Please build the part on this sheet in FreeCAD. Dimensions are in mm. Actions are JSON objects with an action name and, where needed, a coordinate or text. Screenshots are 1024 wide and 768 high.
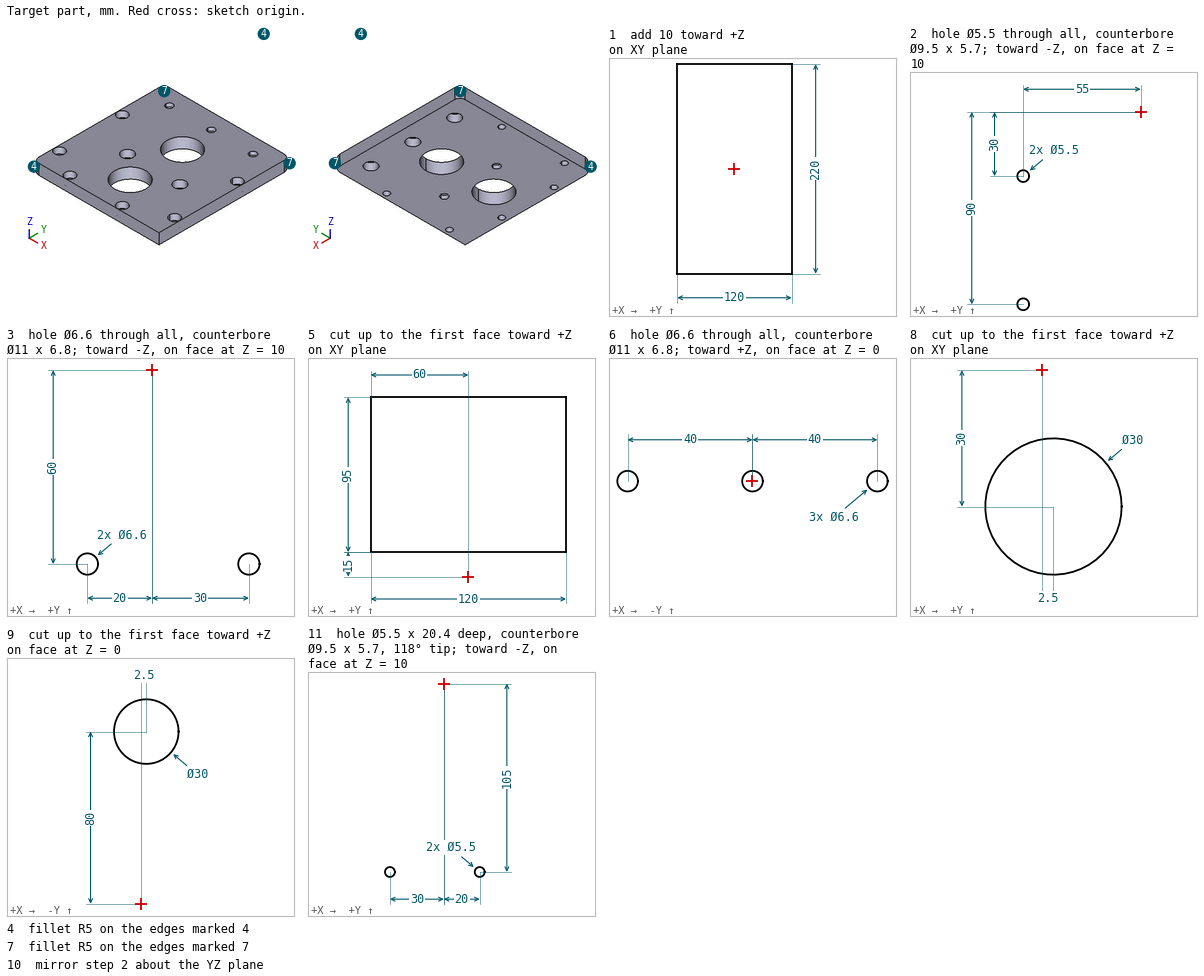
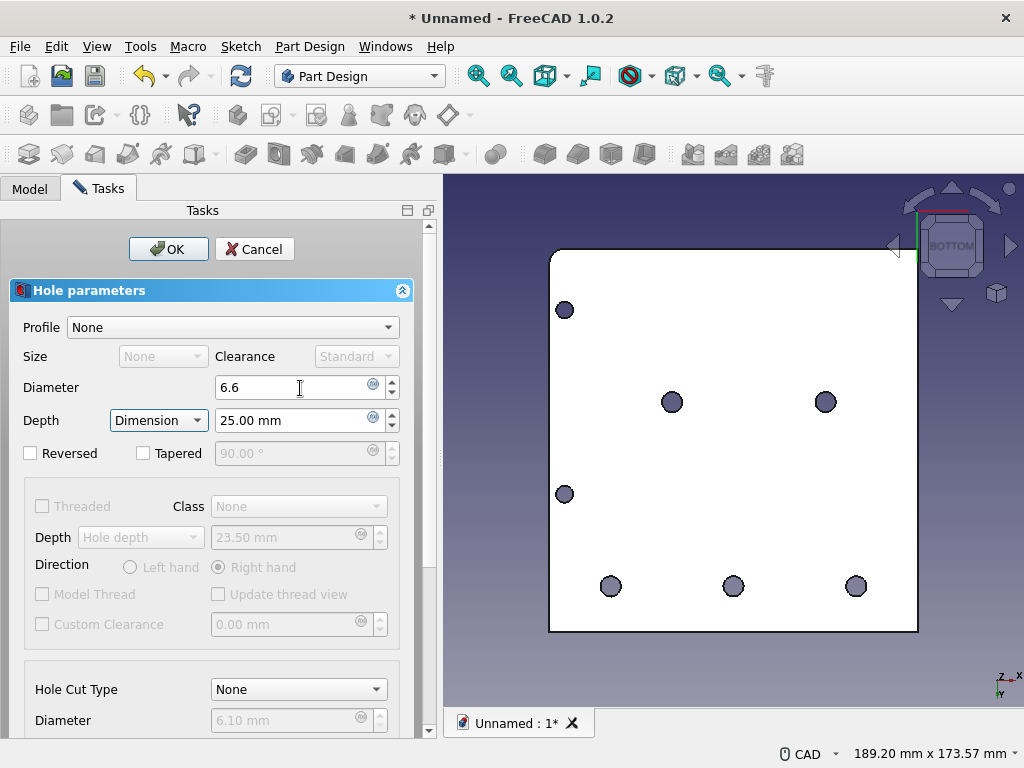
{"action": "left_click", "coordinate": [160, 420]}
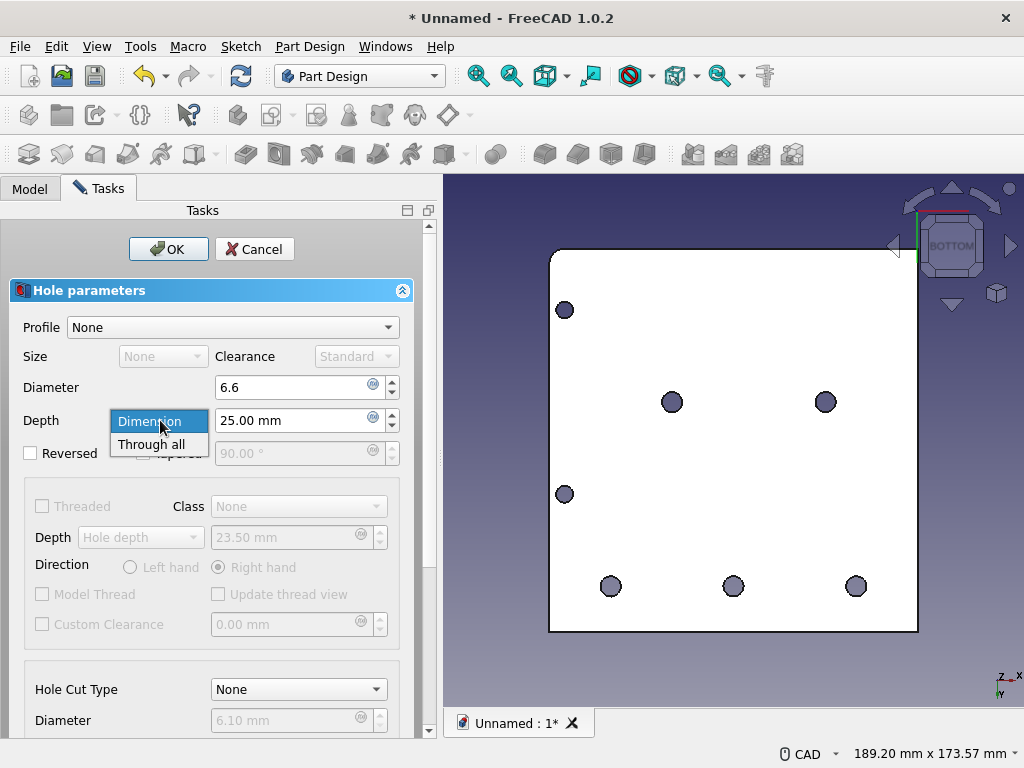
{"action": "left_click", "coordinate": [158, 444]}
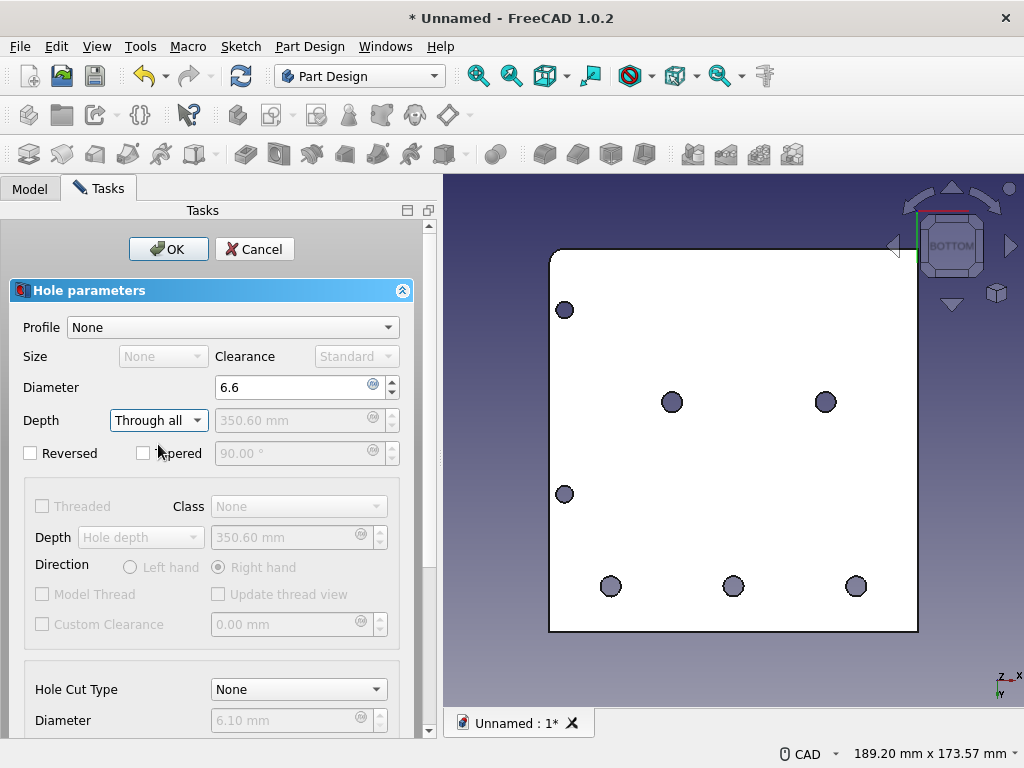
{"action": "left_click", "coordinate": [300, 690]}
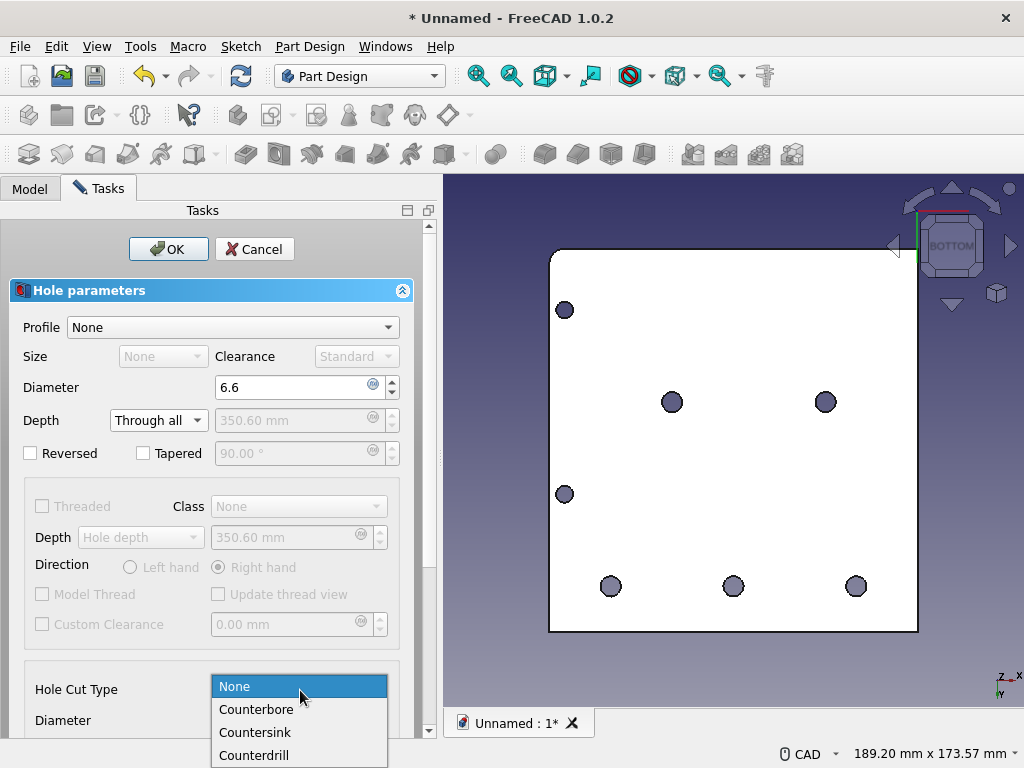
{"action": "left_click", "coordinate": [298, 710]}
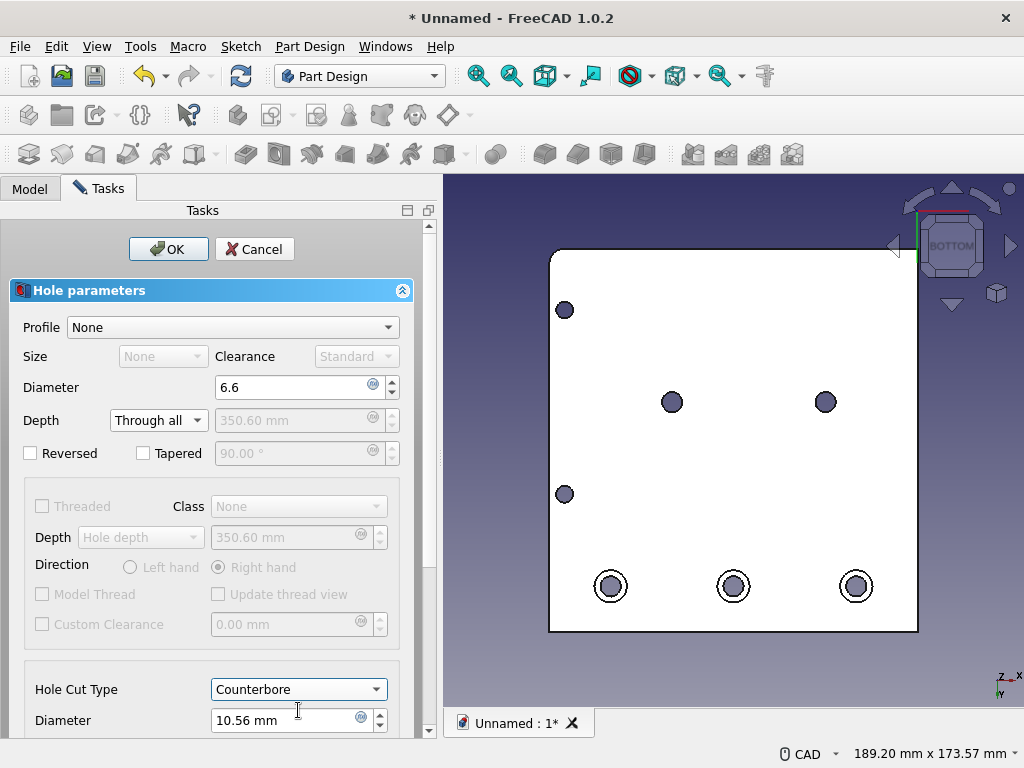
{"action": "triple_click", "coordinate": [292, 720]}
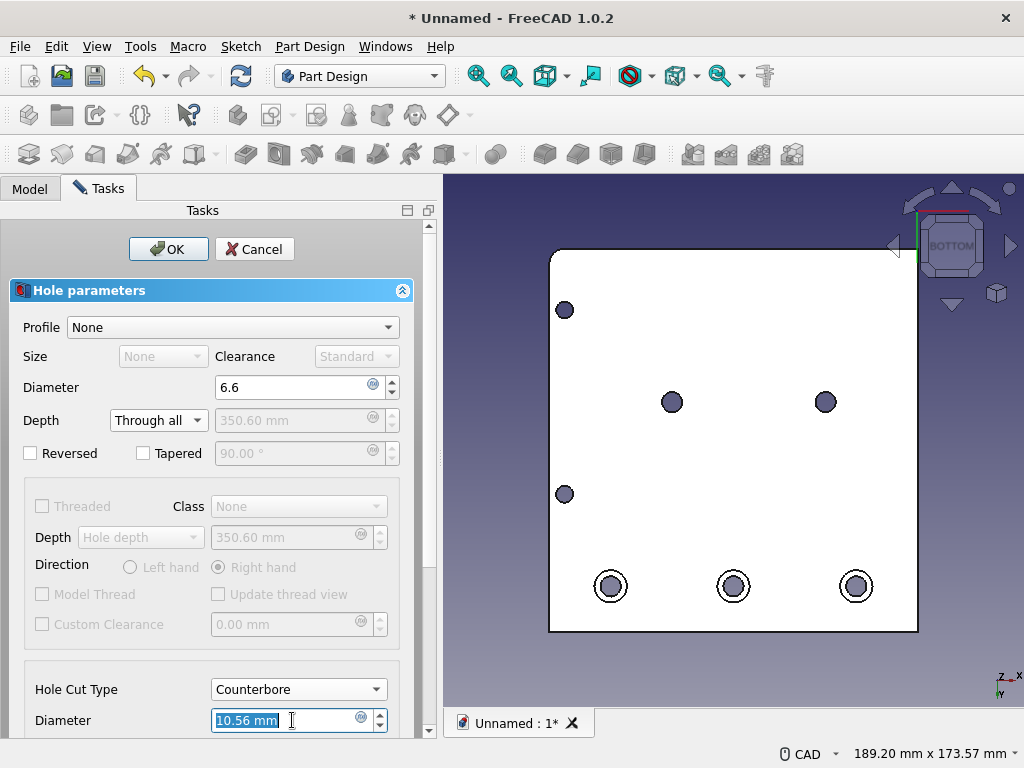
{"action": "type", "text": "11"}
{"action": "key", "text": "Tab"}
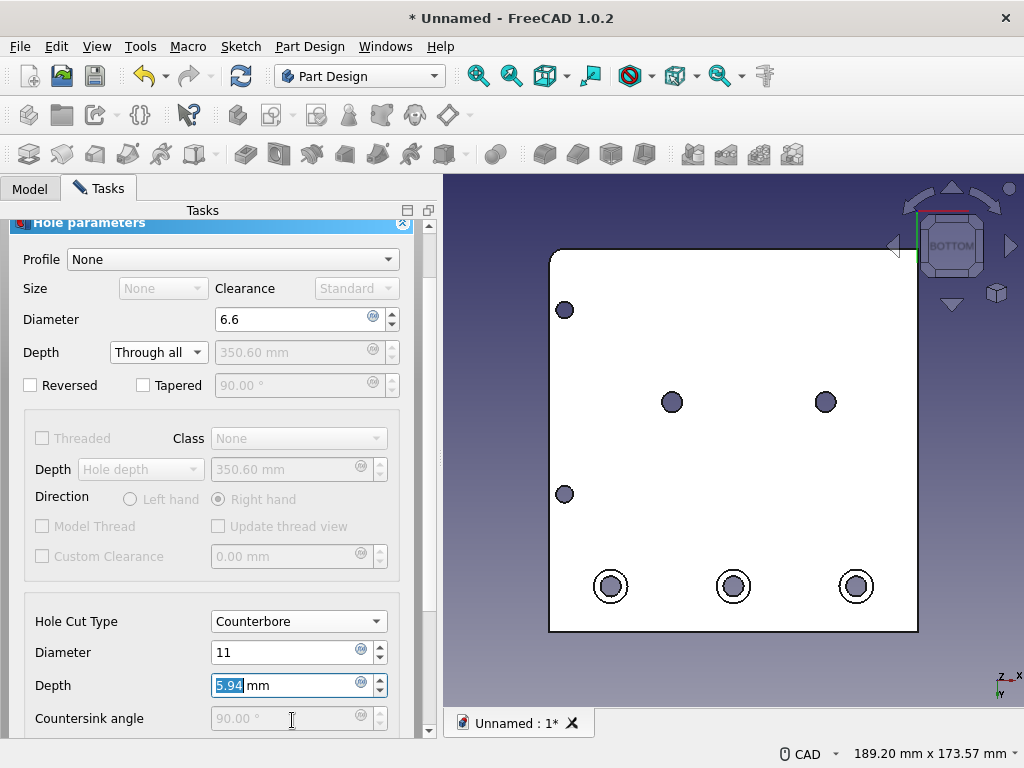
{"action": "type", "text": "6.8"}
{"action": "key", "text": "Tab"}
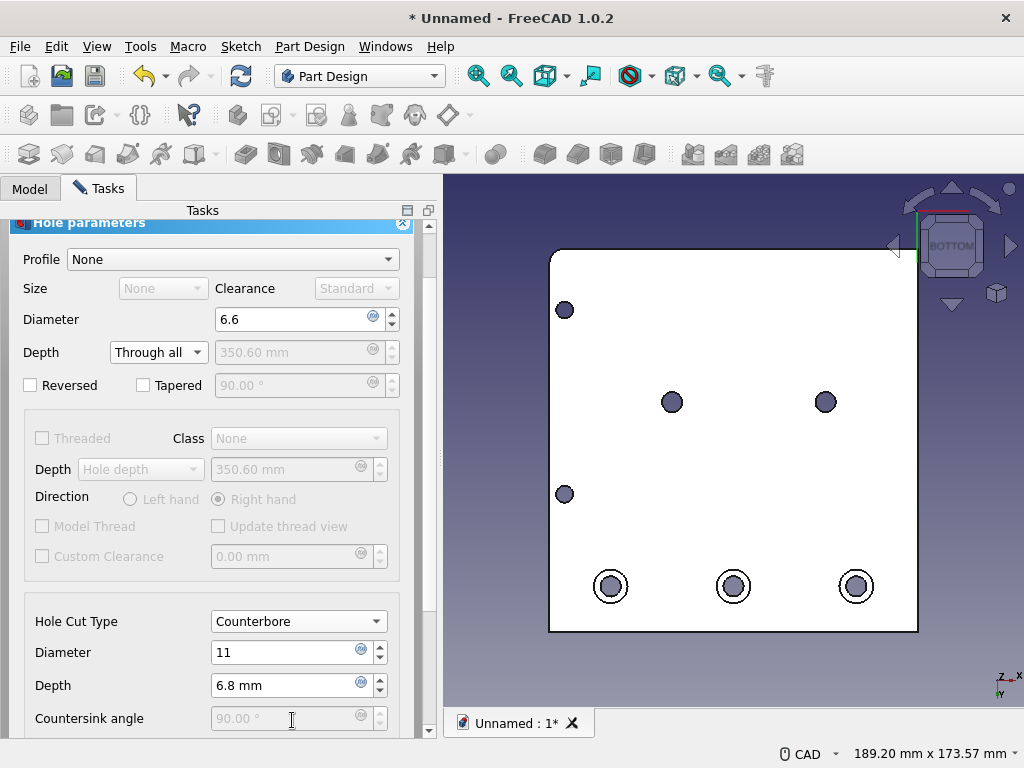
{"action": "scroll", "coordinate": [429, 479], "scroll_direction": "up", "scroll_amount": 2}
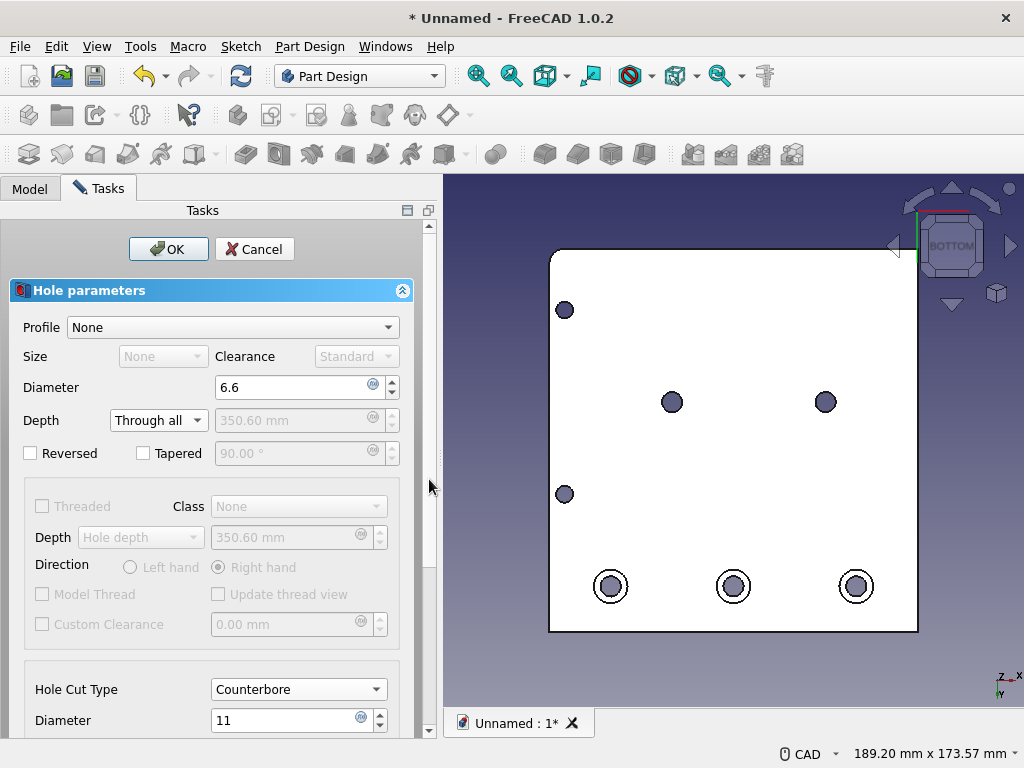
{"action": "left_click", "coordinate": [169, 249]}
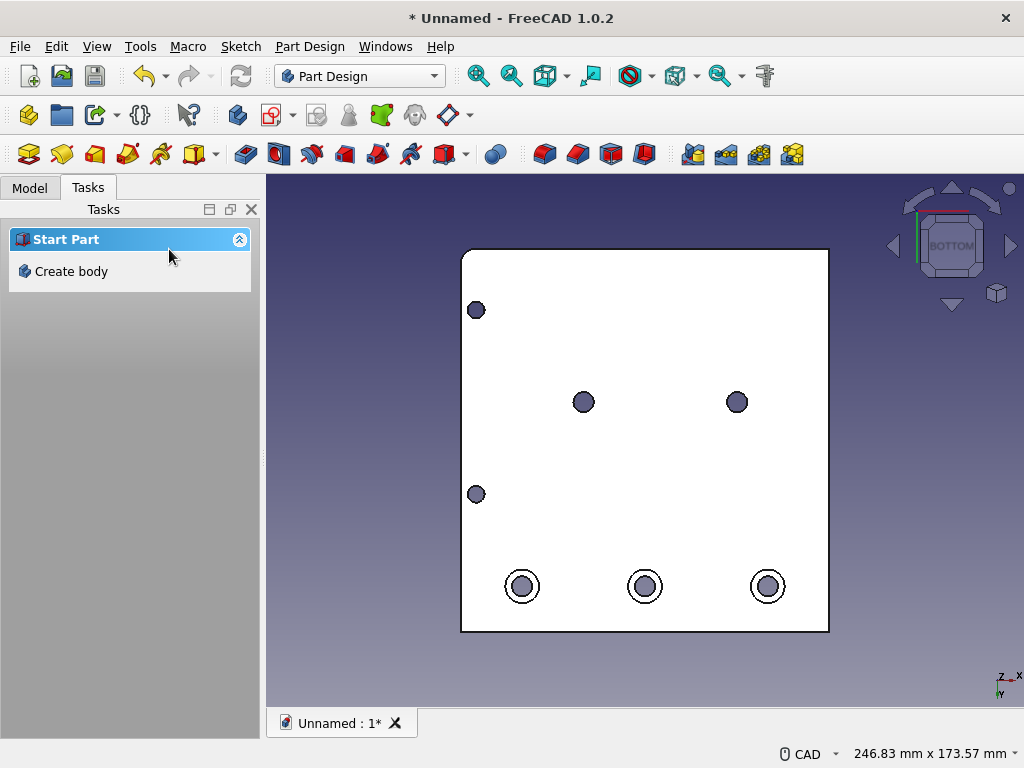
{"action": "key", "text": "0"}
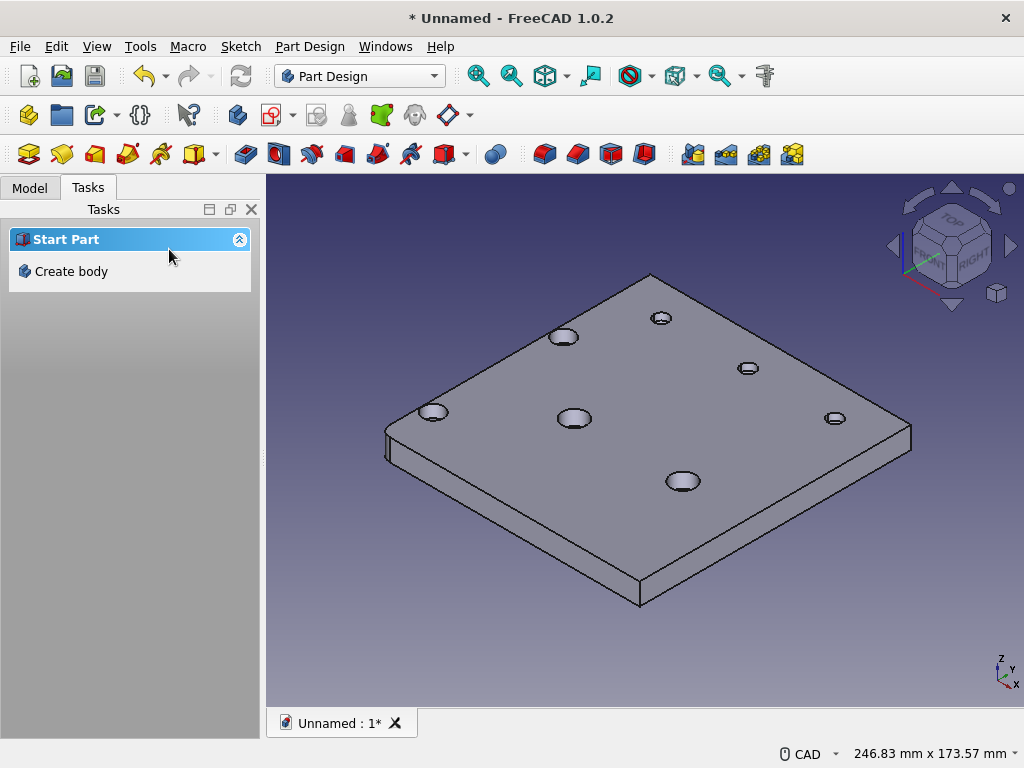
{"action": "key", "text": "2"}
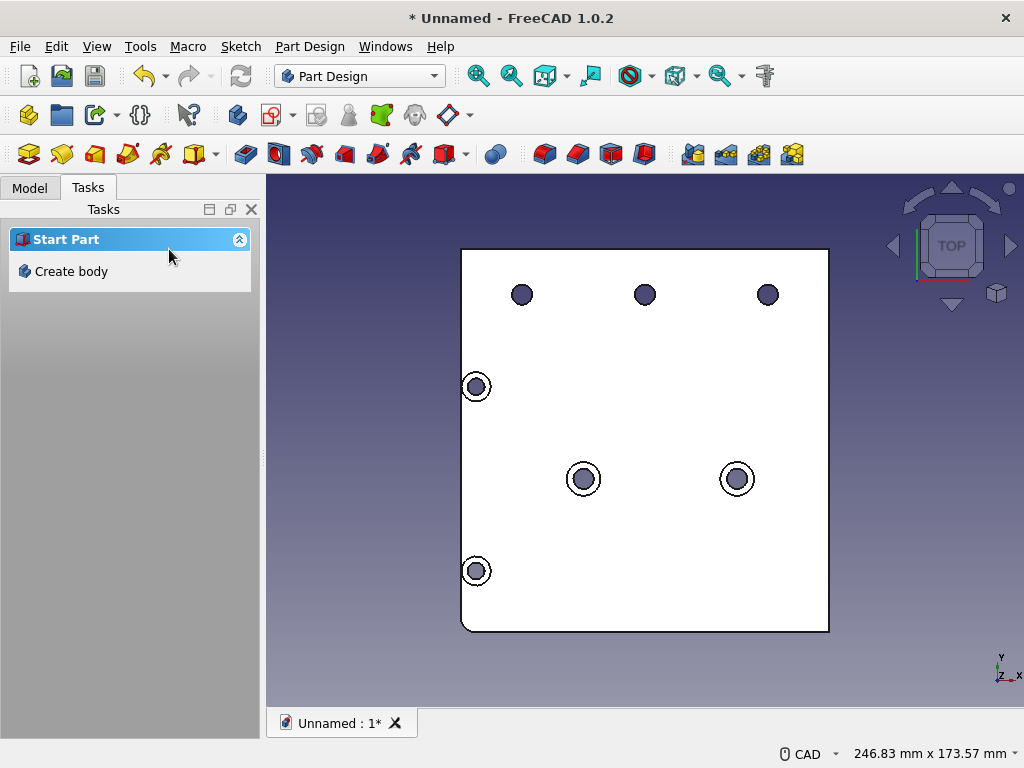
{"action": "key", "text": "1"}